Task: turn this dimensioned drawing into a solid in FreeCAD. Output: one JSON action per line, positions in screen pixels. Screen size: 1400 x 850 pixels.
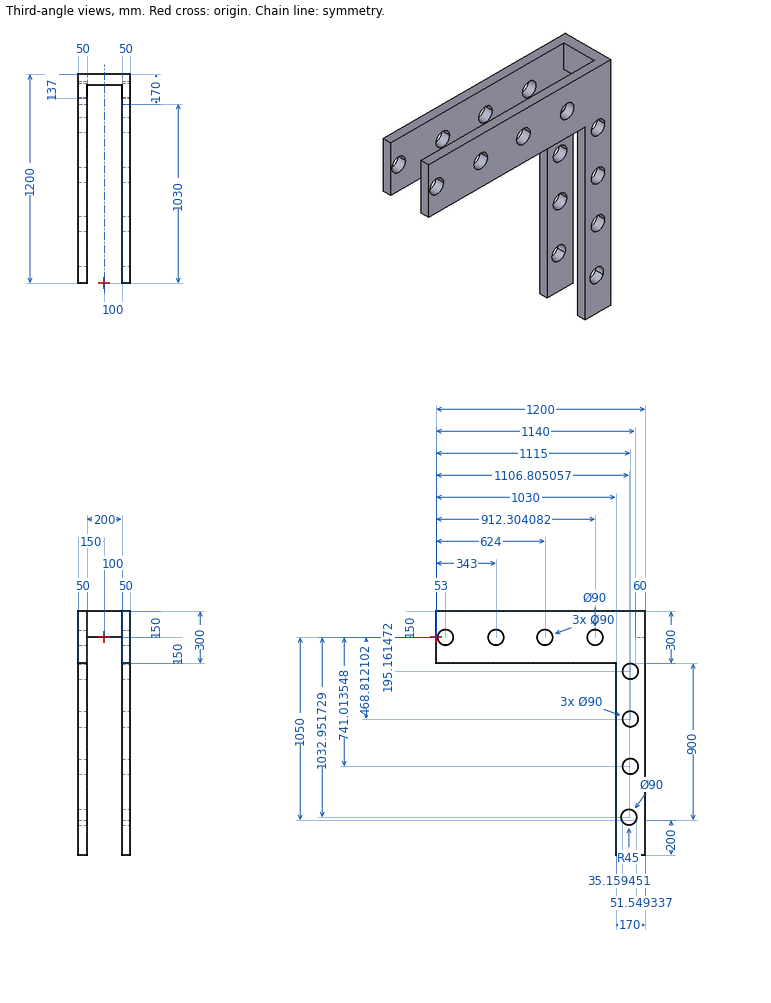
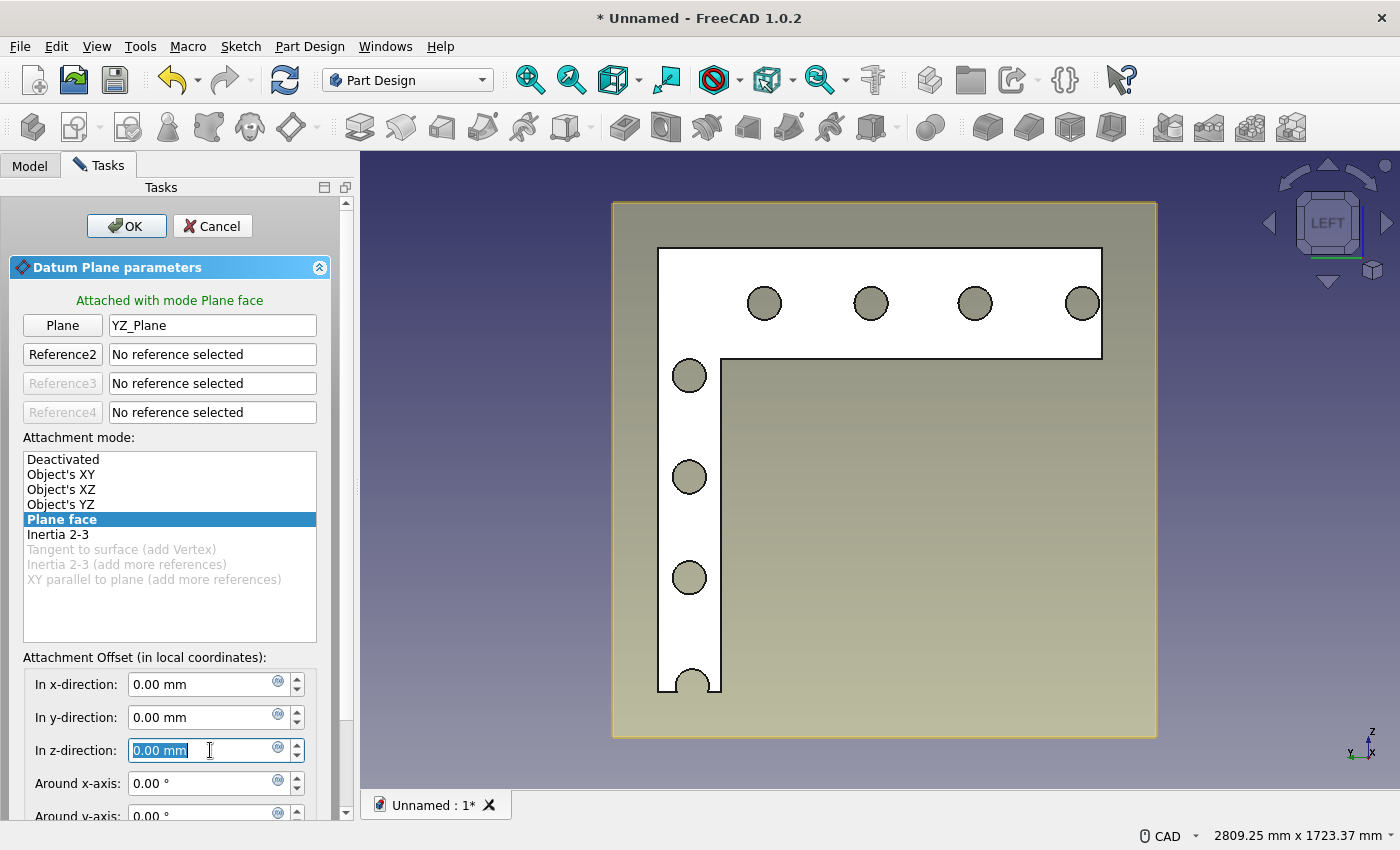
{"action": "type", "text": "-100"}
{"action": "key", "text": "Tab"}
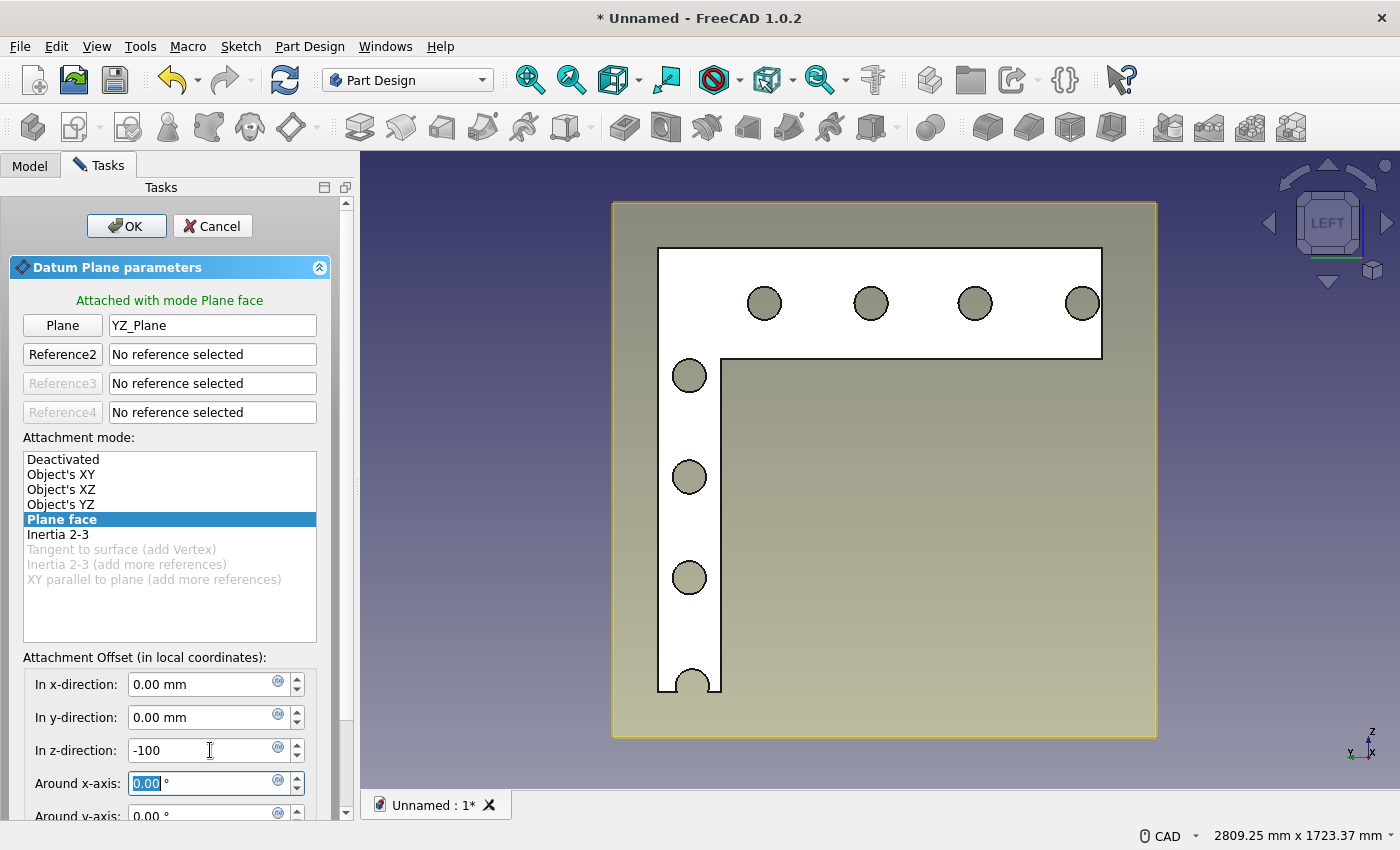
{"action": "left_click", "coordinate": [127, 226]}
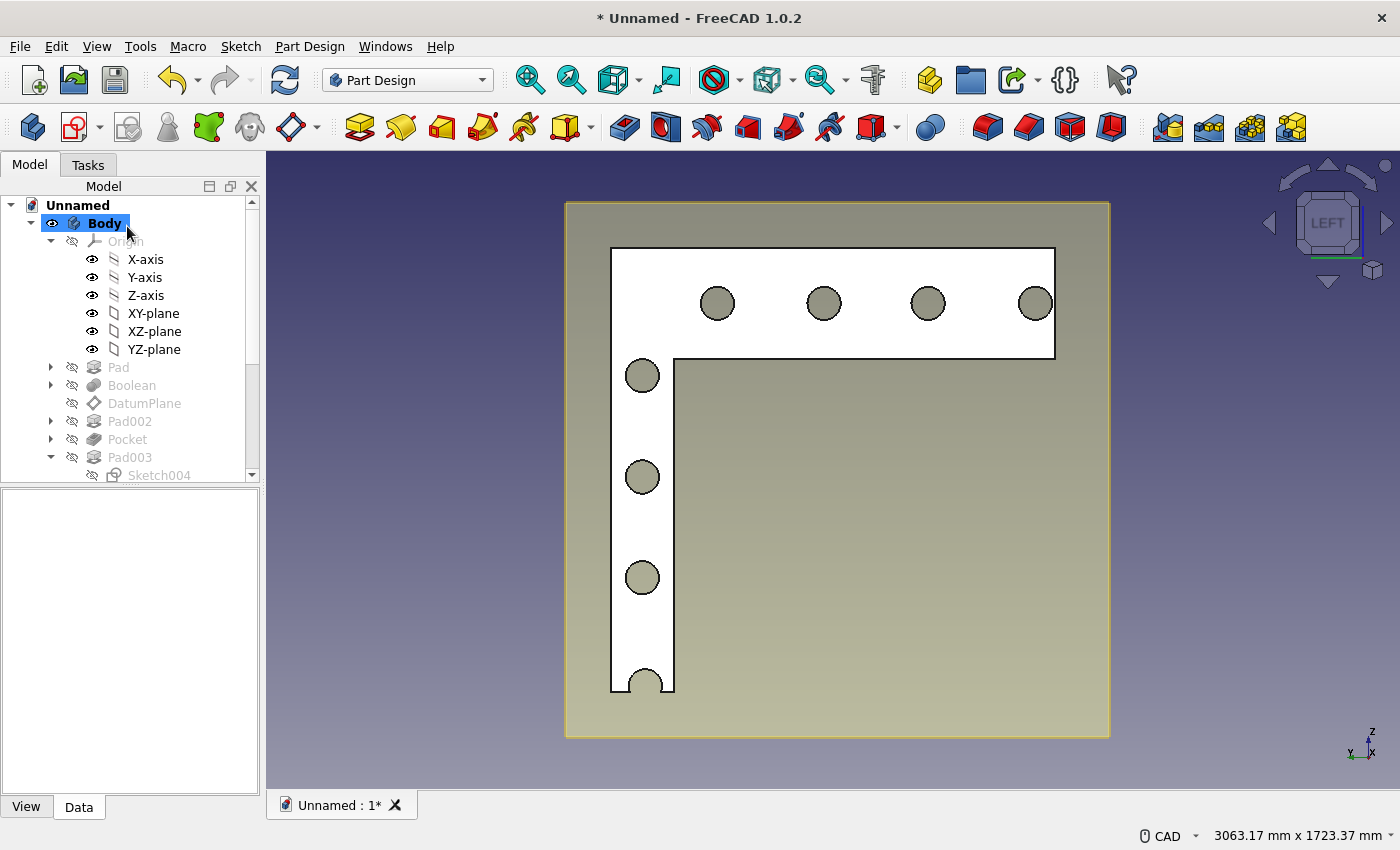
{"action": "scroll", "coordinate": [101, 345], "scroll_direction": "down", "scroll_amount": 3}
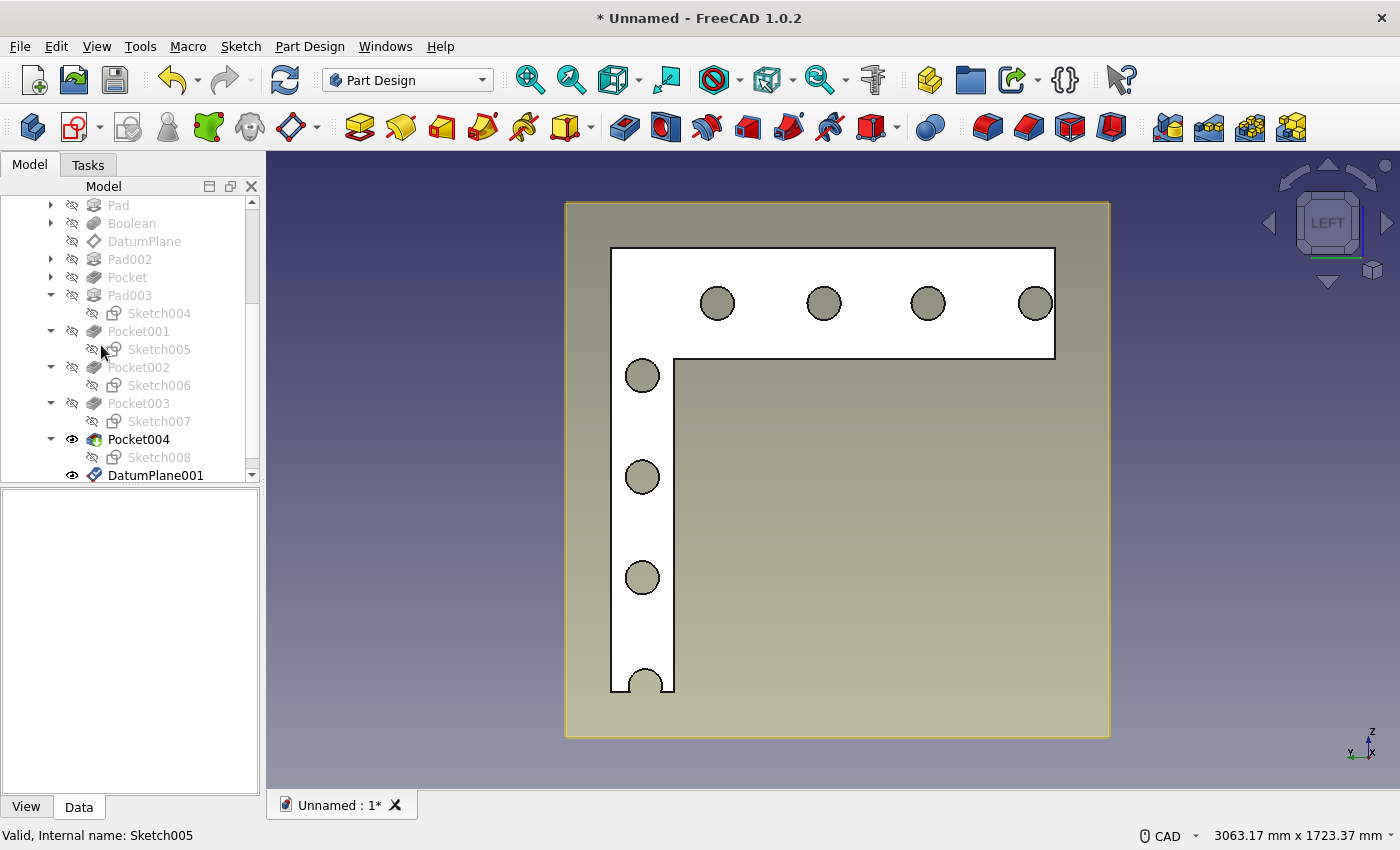
{"action": "left_click", "coordinate": [117, 475]}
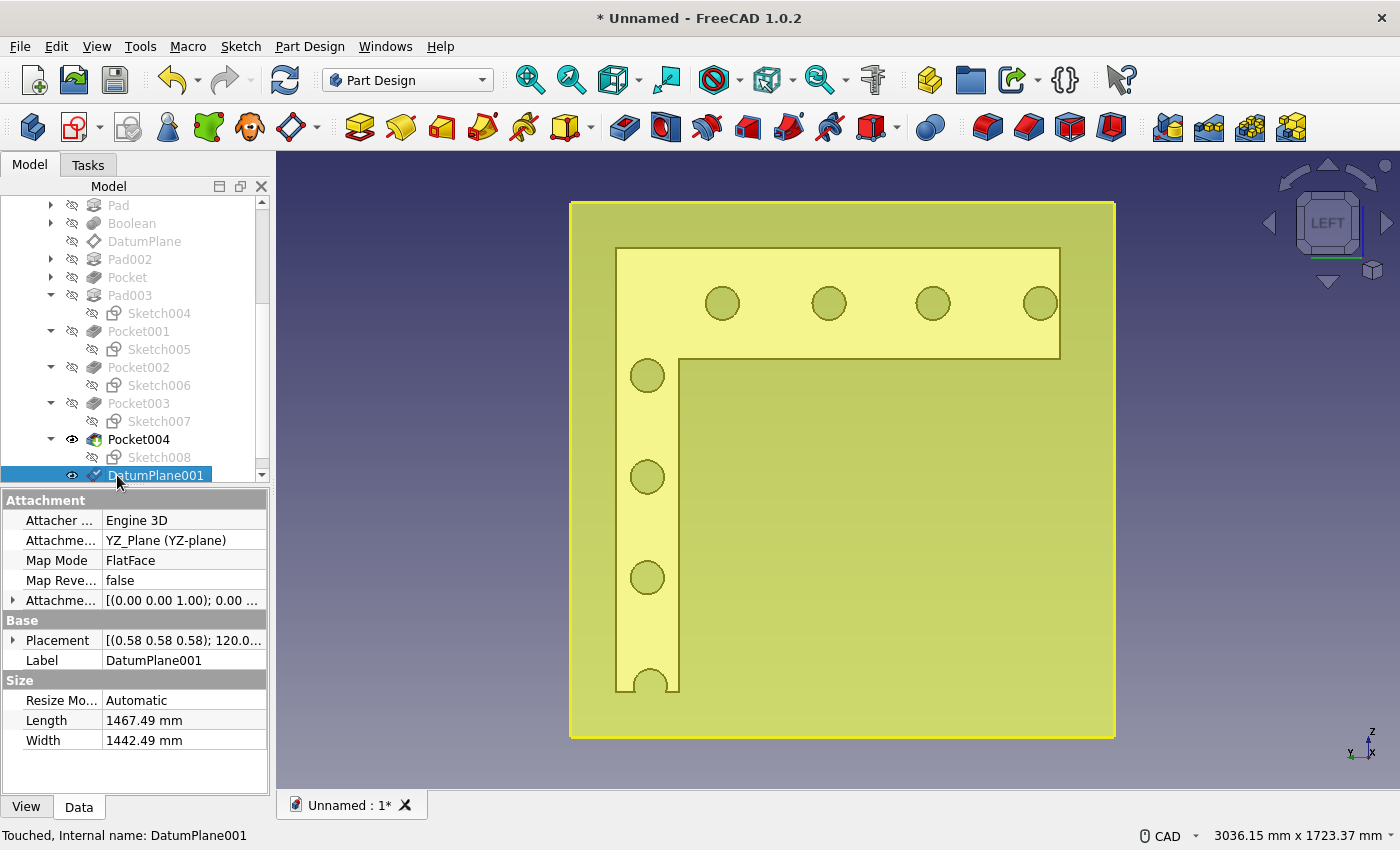
{"action": "left_click", "coordinate": [74, 128]}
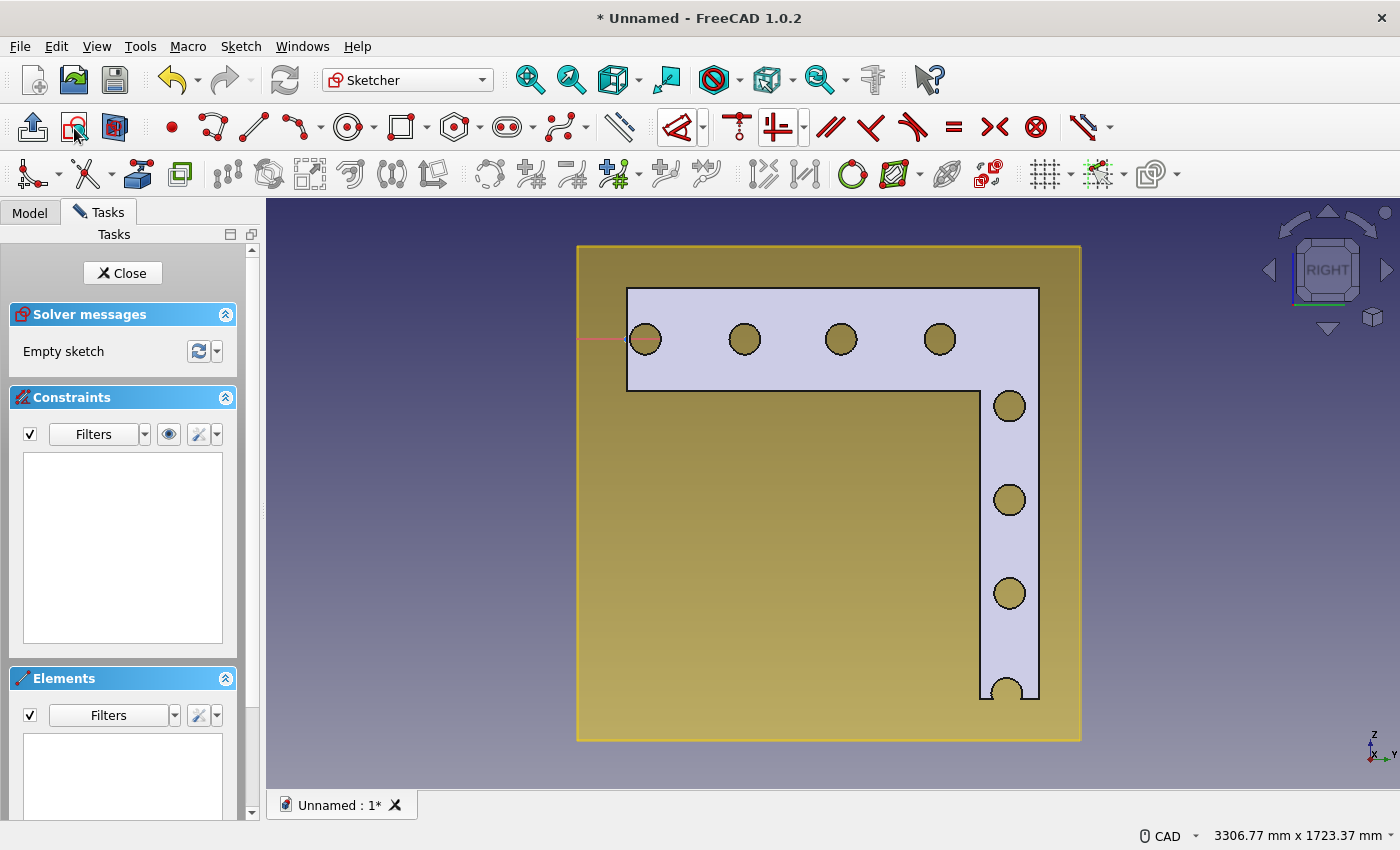
{"action": "left_click", "coordinate": [115, 128]}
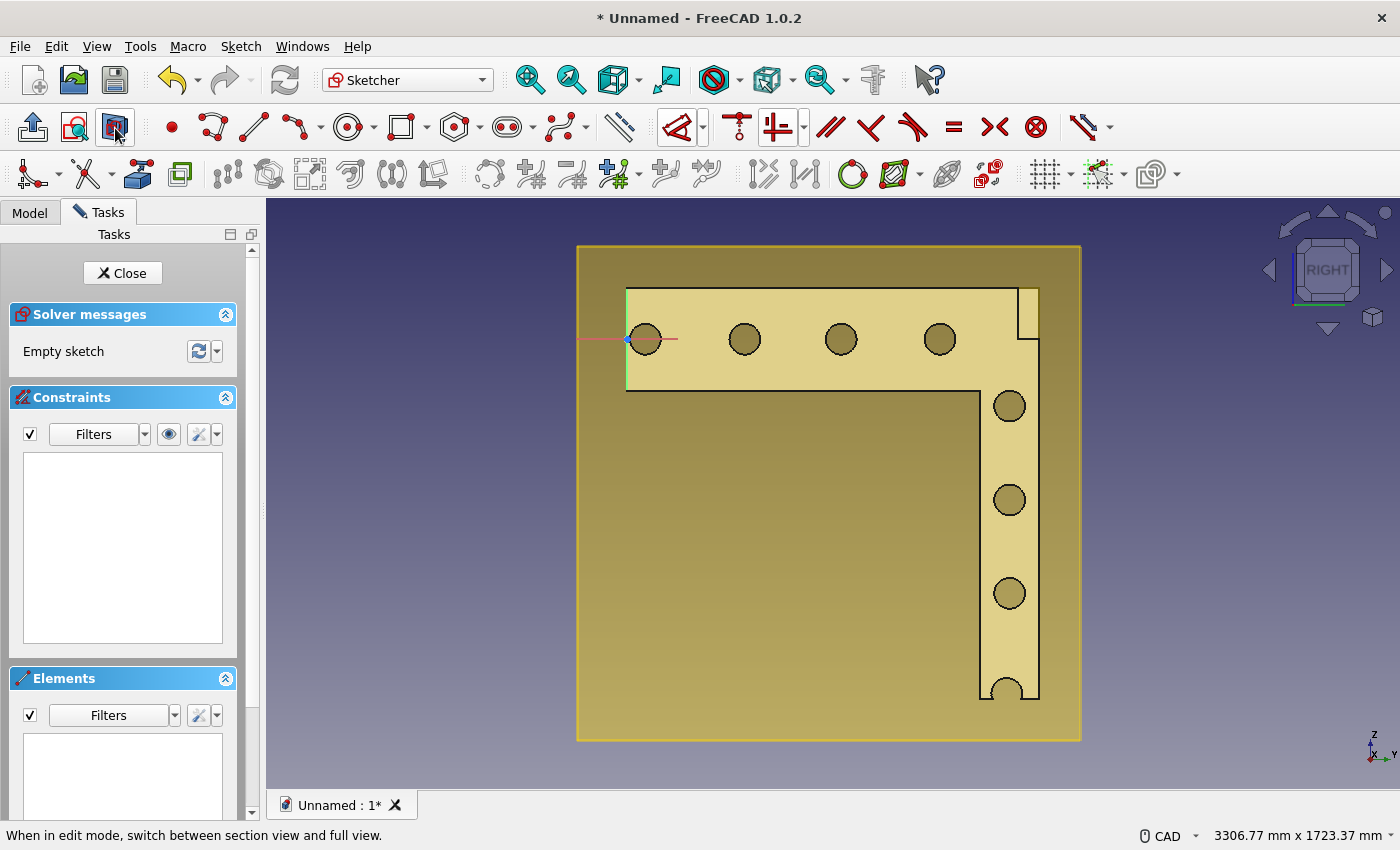
{"action": "scroll", "coordinate": [764, 494], "scroll_direction": "down", "scroll_amount": 5}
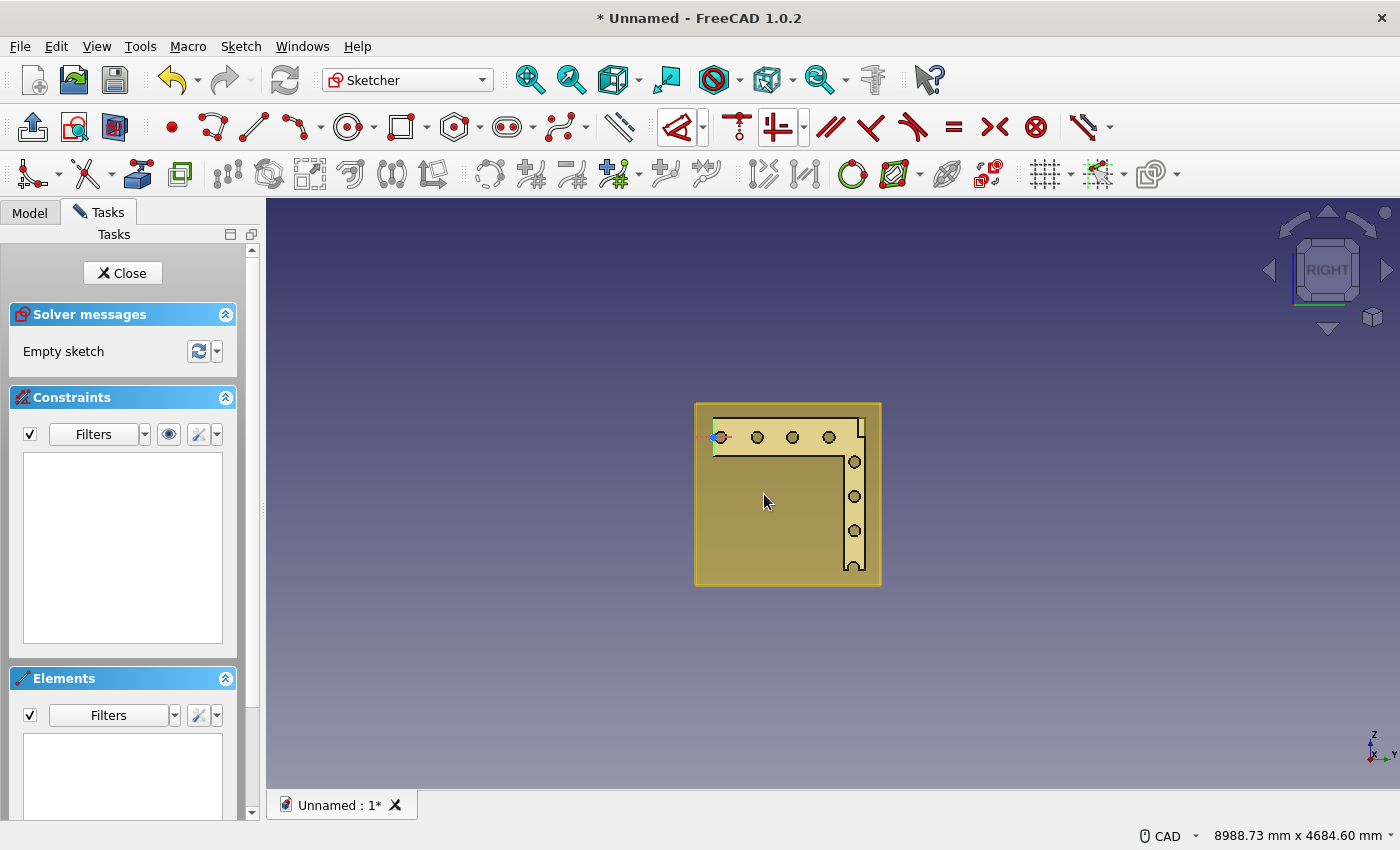
{"action": "scroll", "coordinate": [860, 588], "scroll_direction": "up", "scroll_amount": 14}